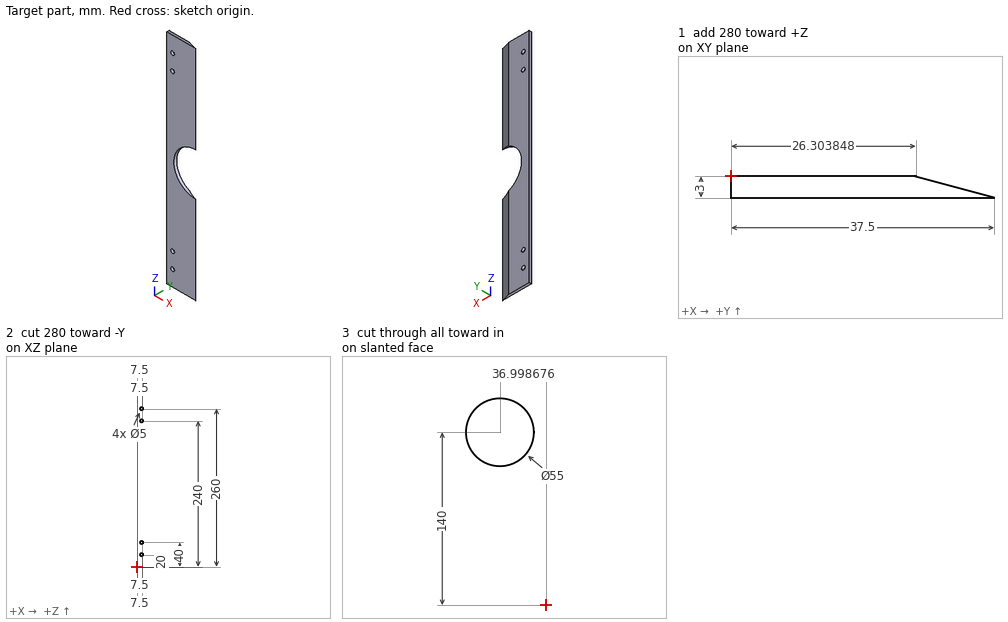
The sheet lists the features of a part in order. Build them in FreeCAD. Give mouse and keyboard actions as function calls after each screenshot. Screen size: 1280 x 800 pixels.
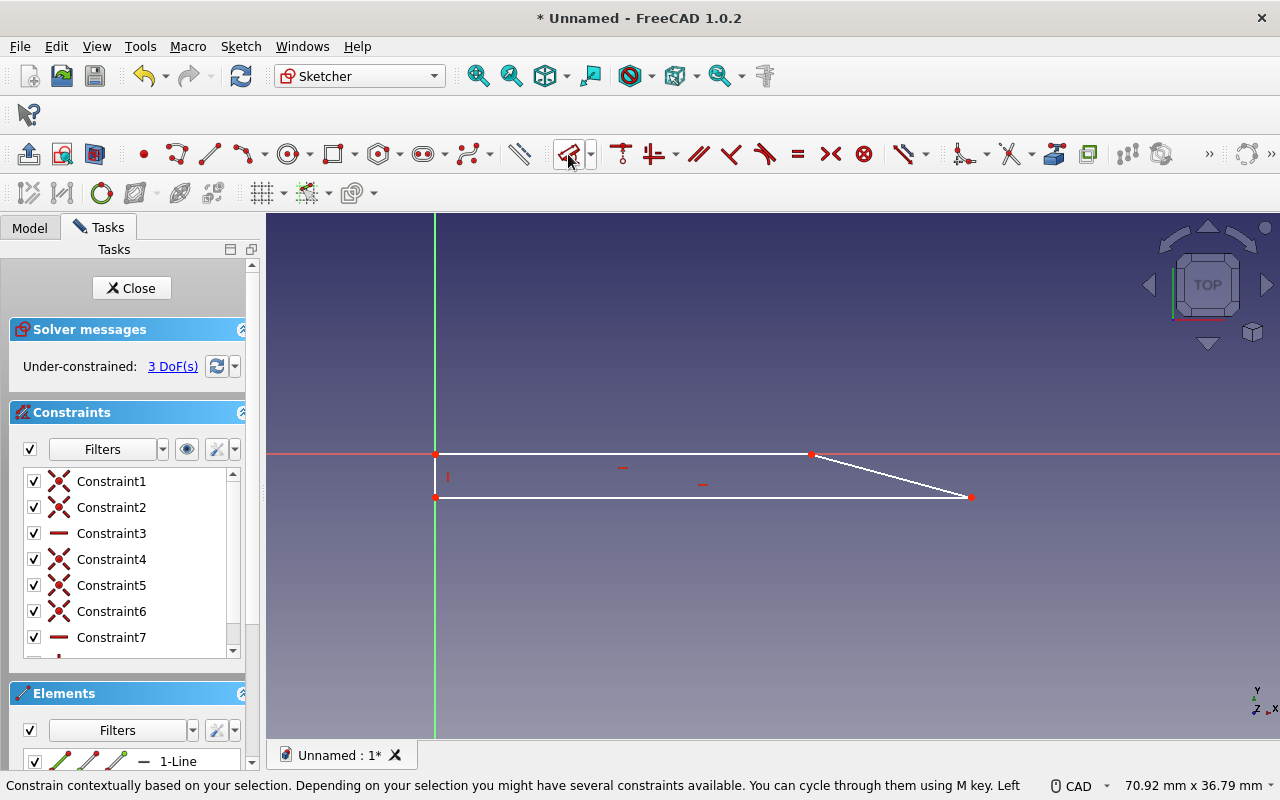
click(435, 468)
click(401, 476)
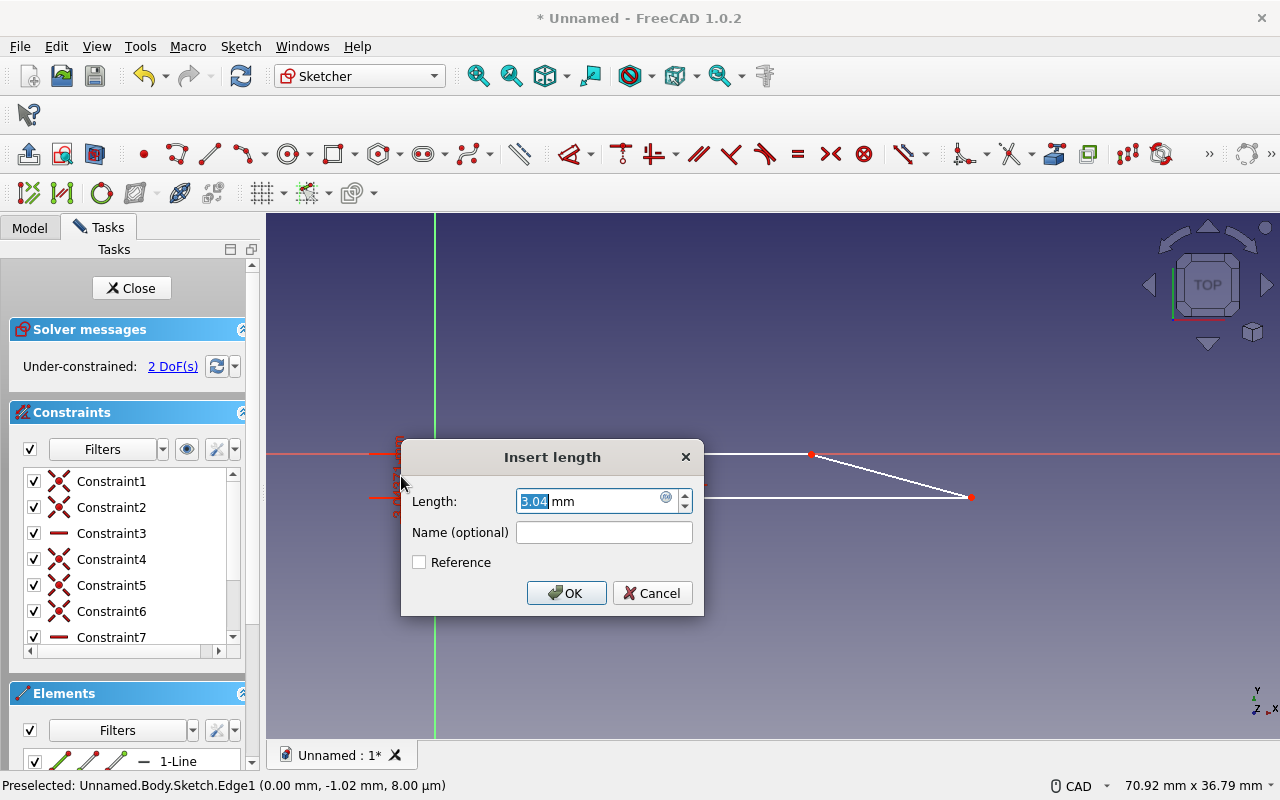
text(3)
key(Return)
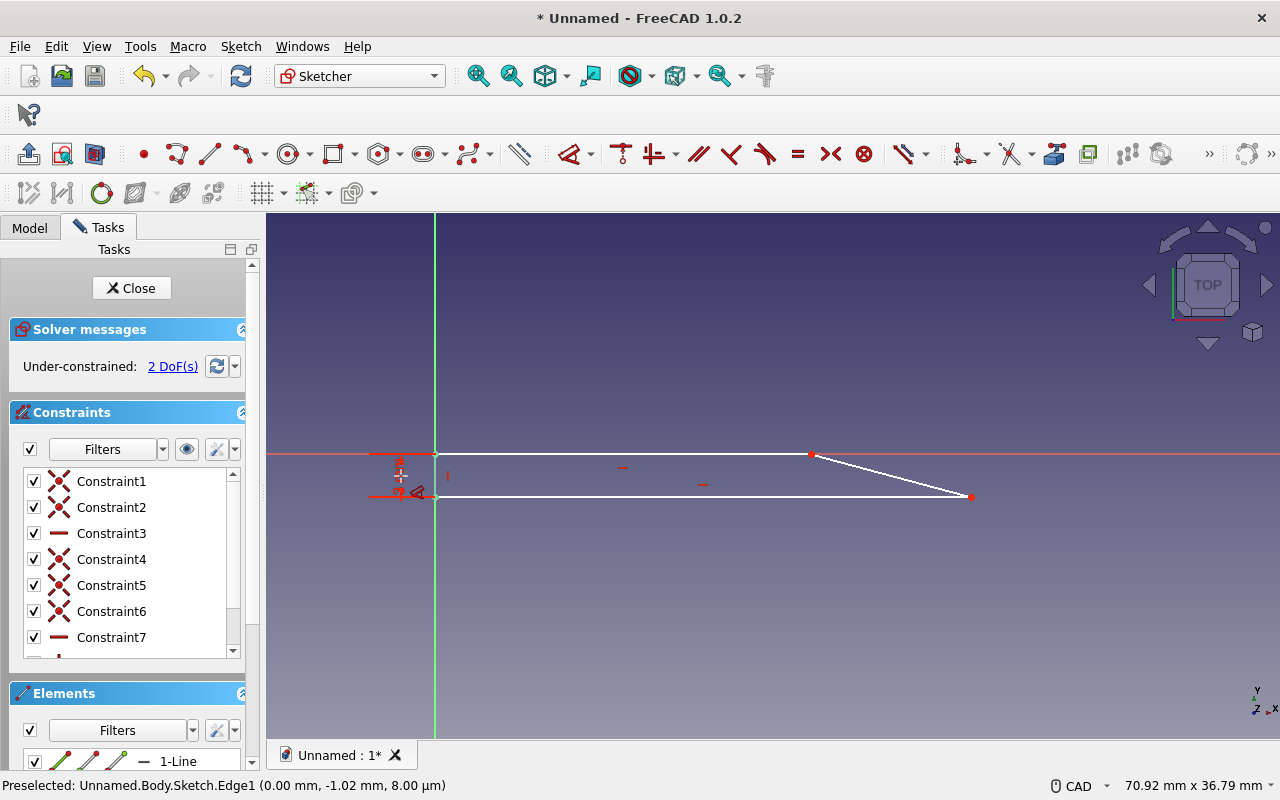
click(596, 497)
click(703, 531)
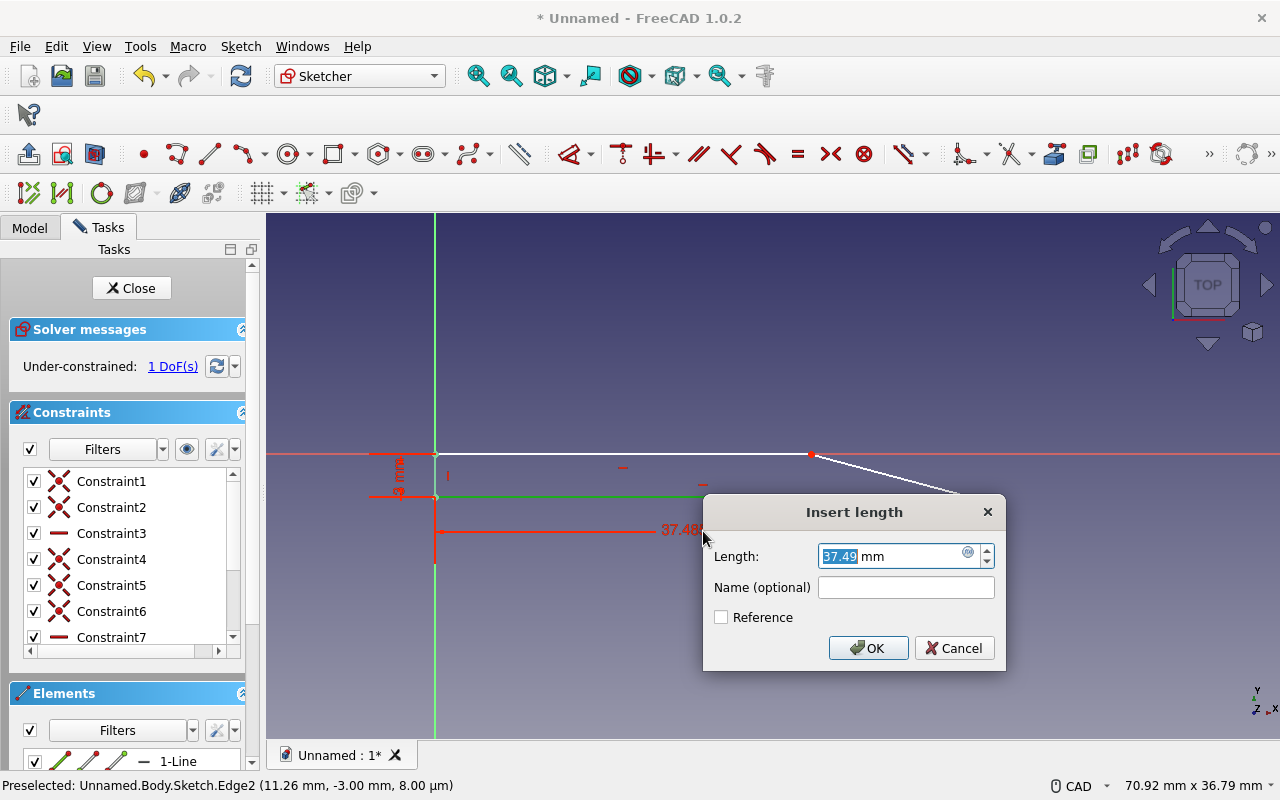
text(37.5)
key(Return)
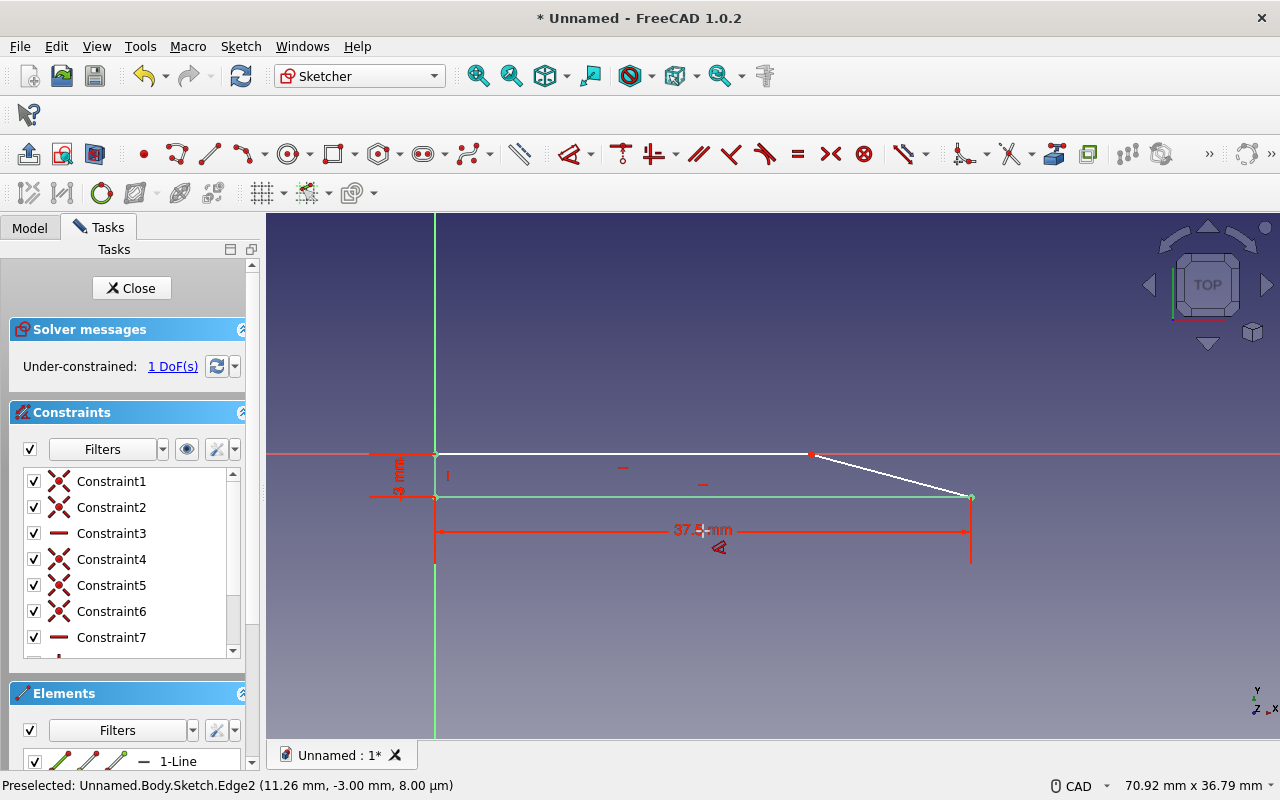
click(698, 454)
click(623, 420)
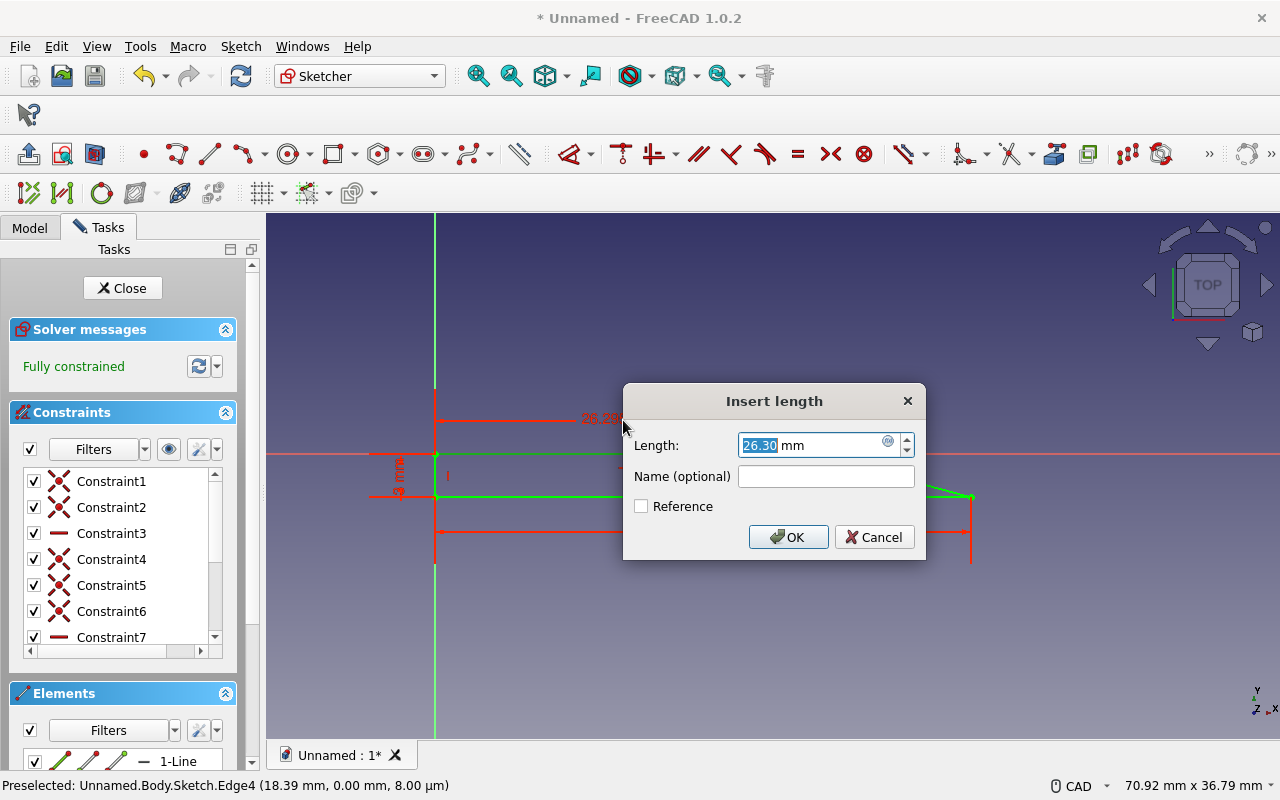
text(26.303848)
key(Return)
key(Escape)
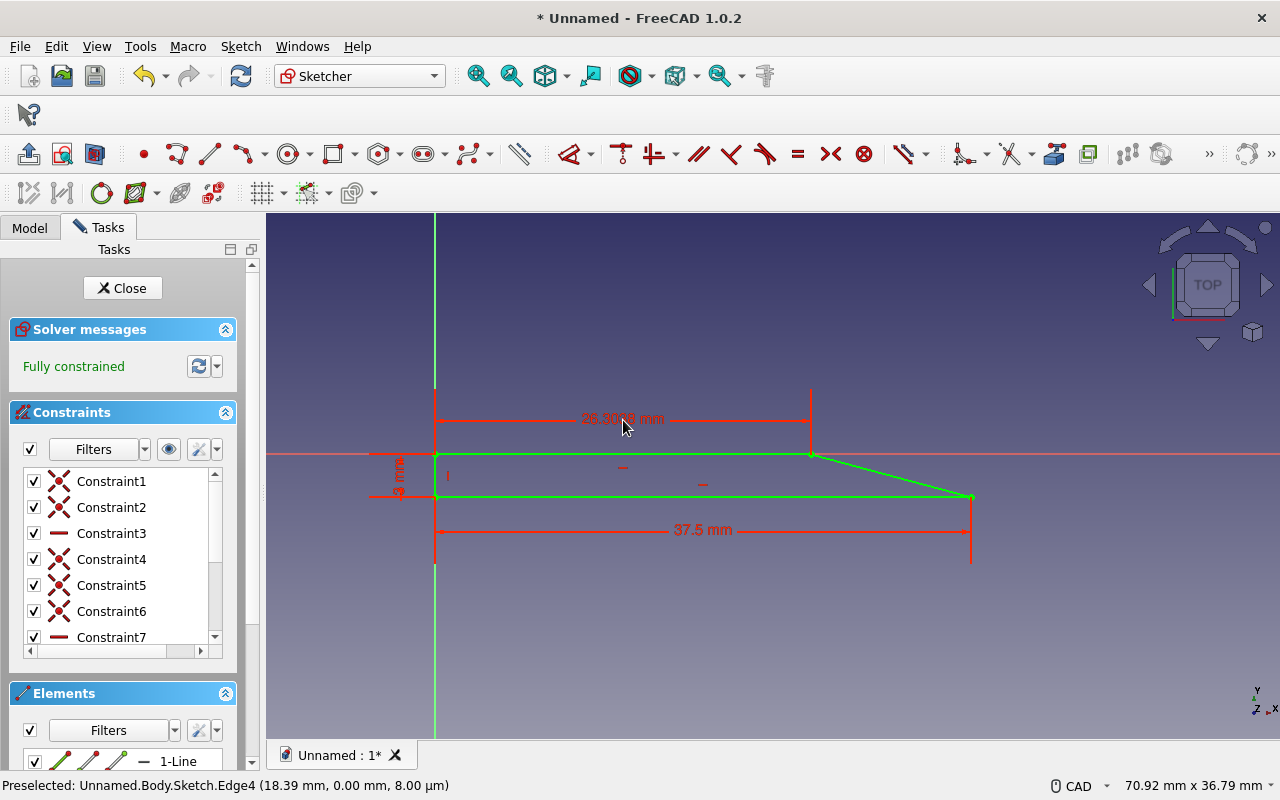
click(123, 288)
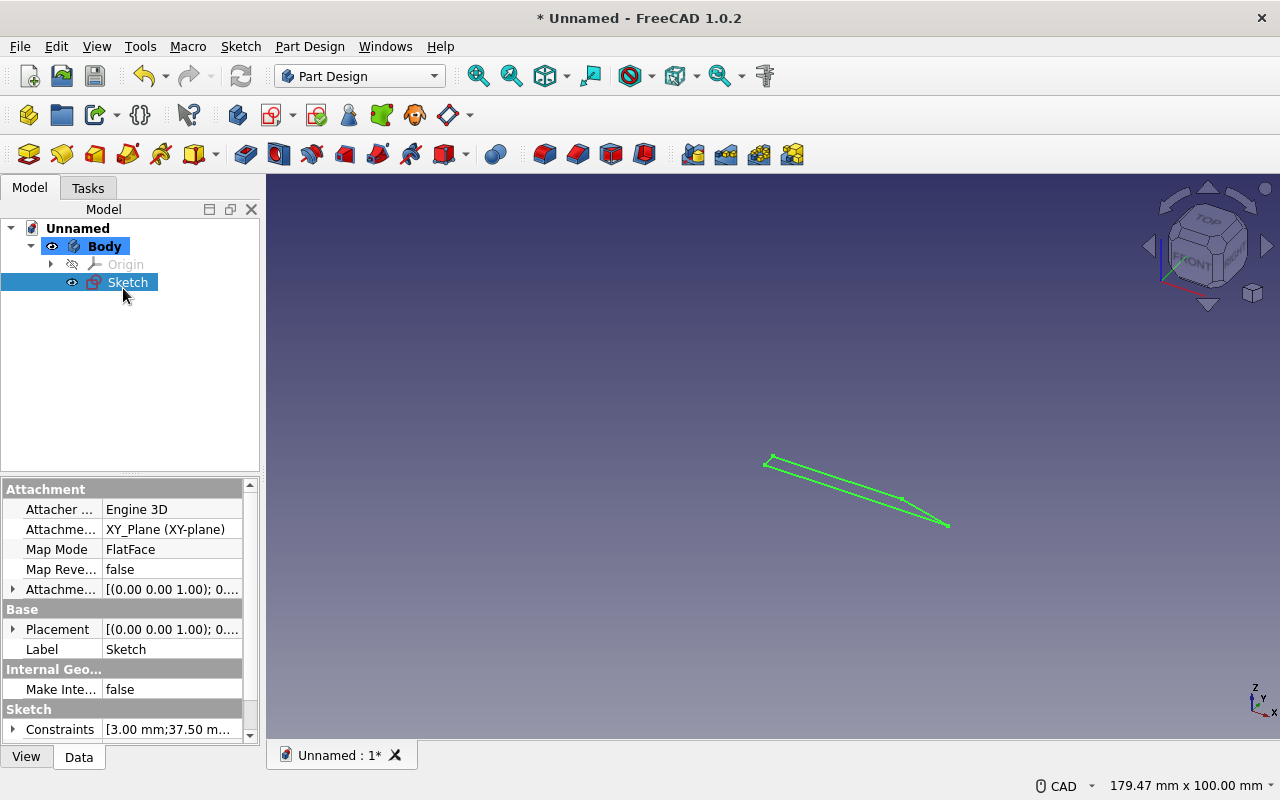
click(29, 154)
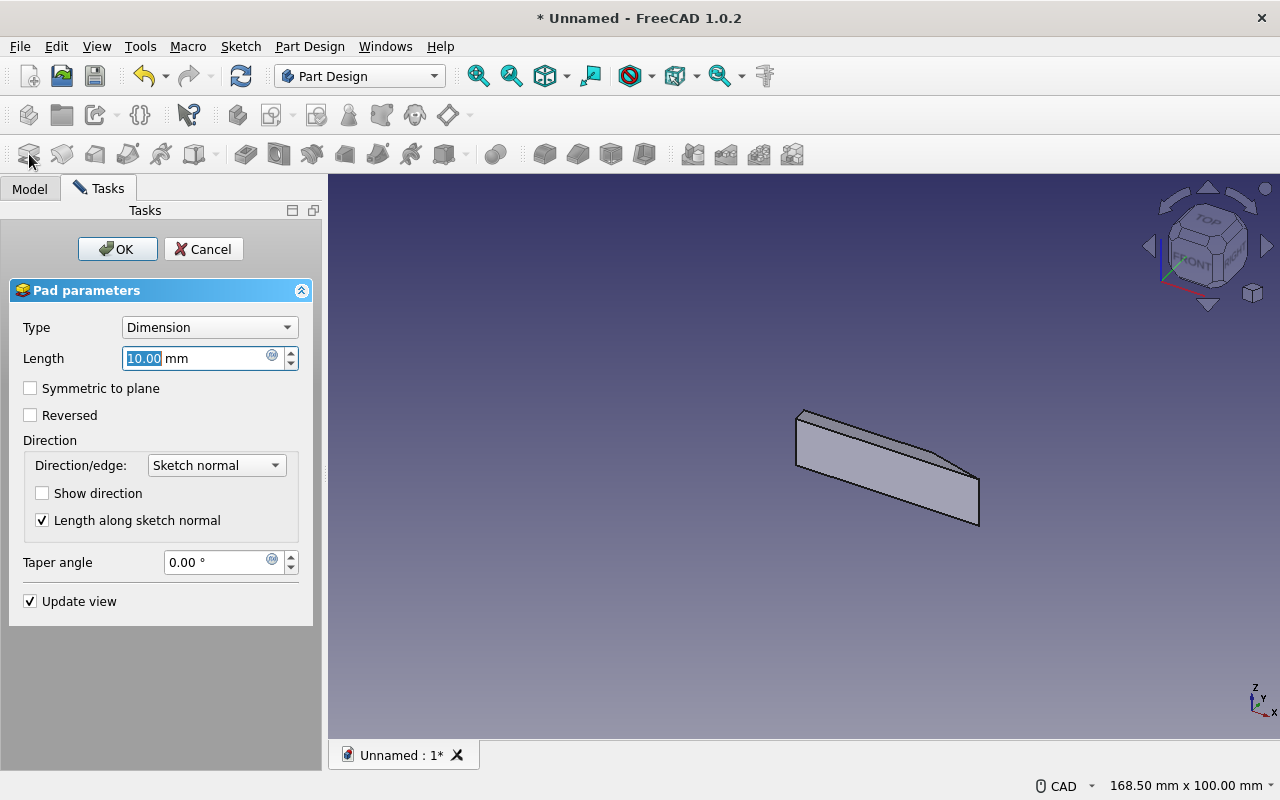
text(280)
key(Tab)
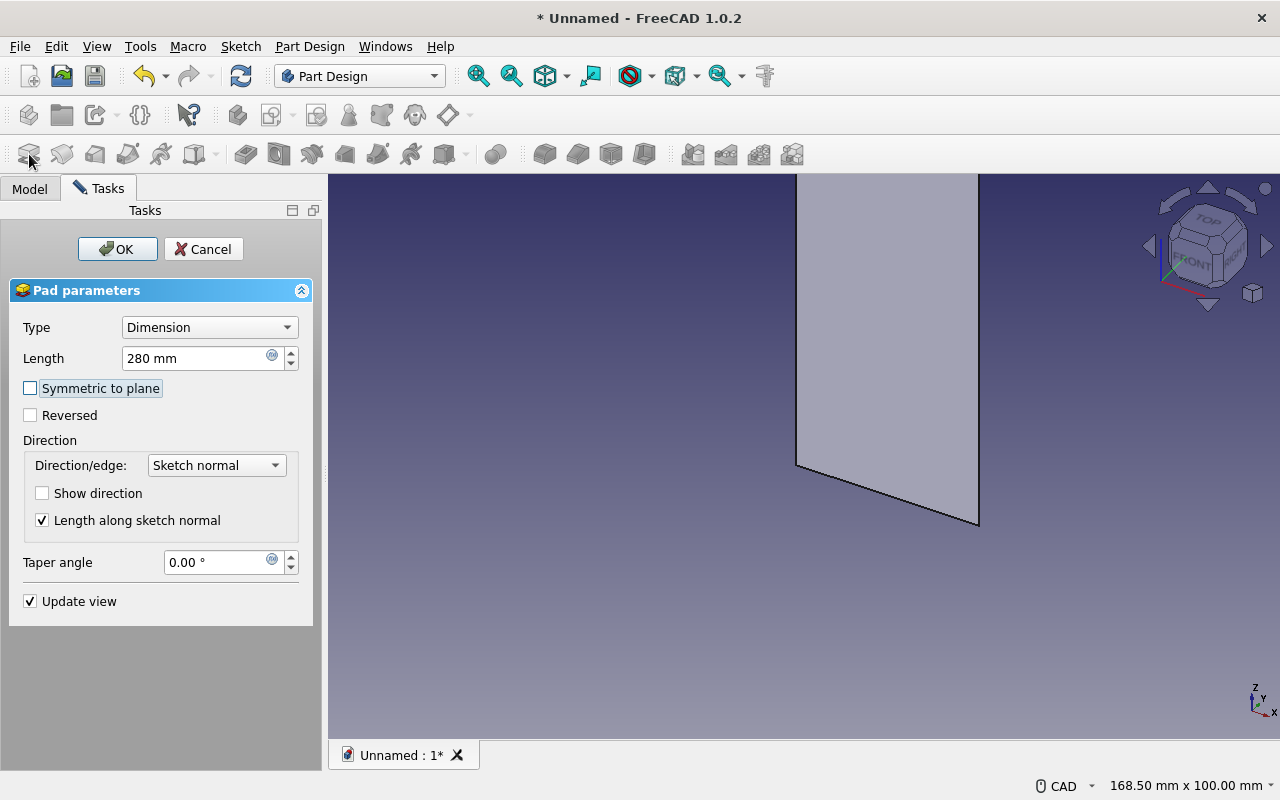
click(118, 249)